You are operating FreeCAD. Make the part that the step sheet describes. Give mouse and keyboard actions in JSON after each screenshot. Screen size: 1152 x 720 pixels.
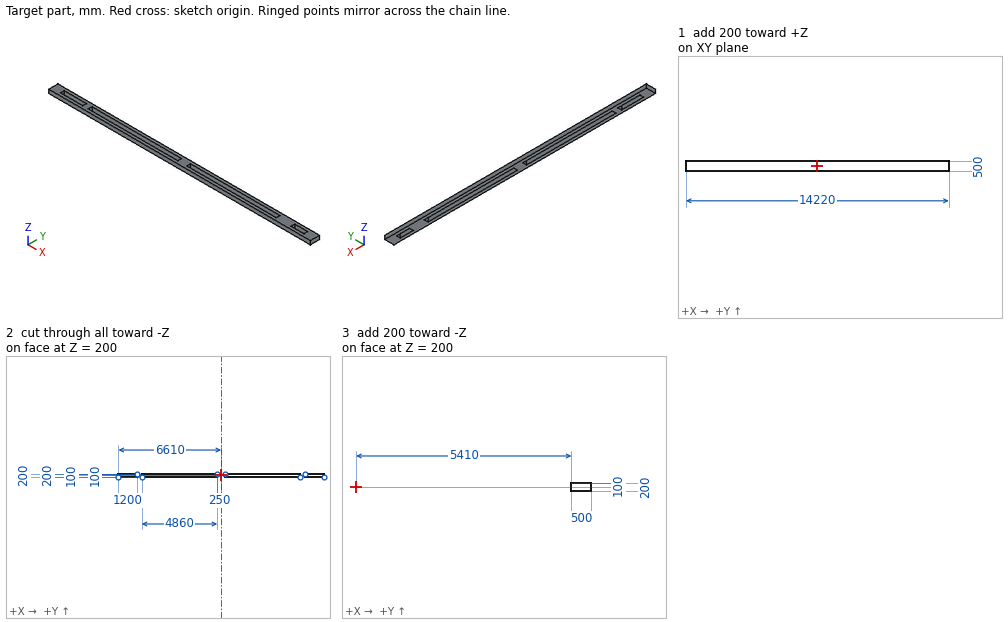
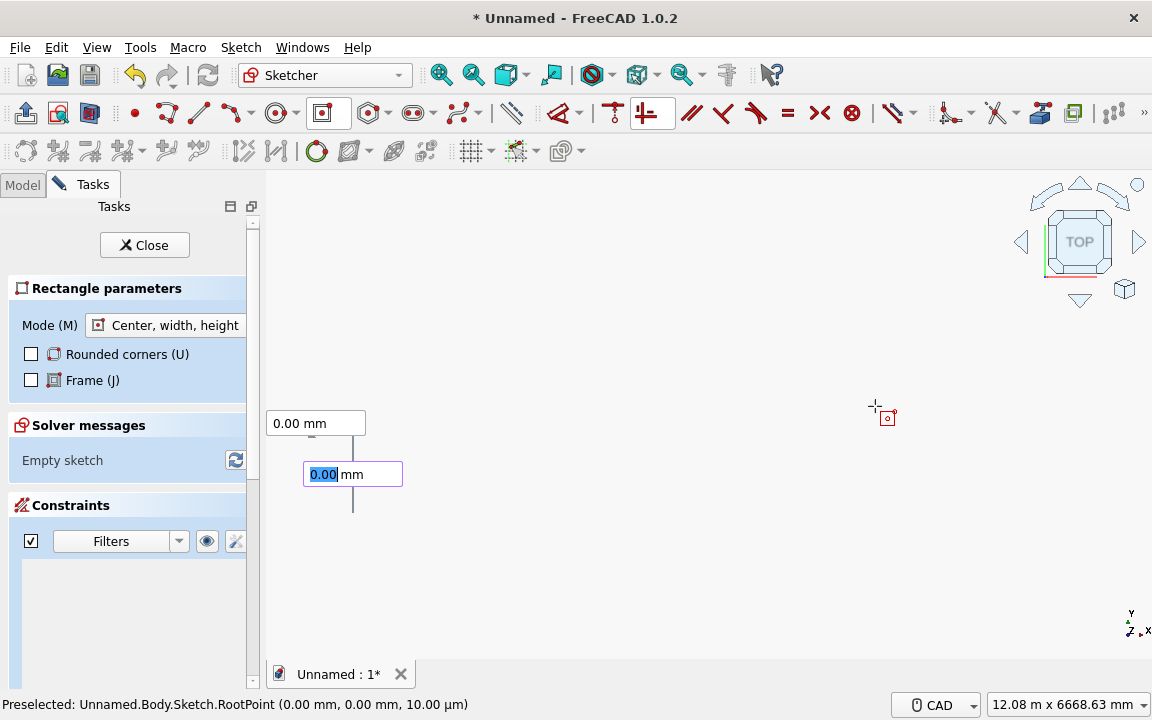
{"action": "left_click", "coordinate": [874, 406]}
{"action": "key", "text": "Escape"}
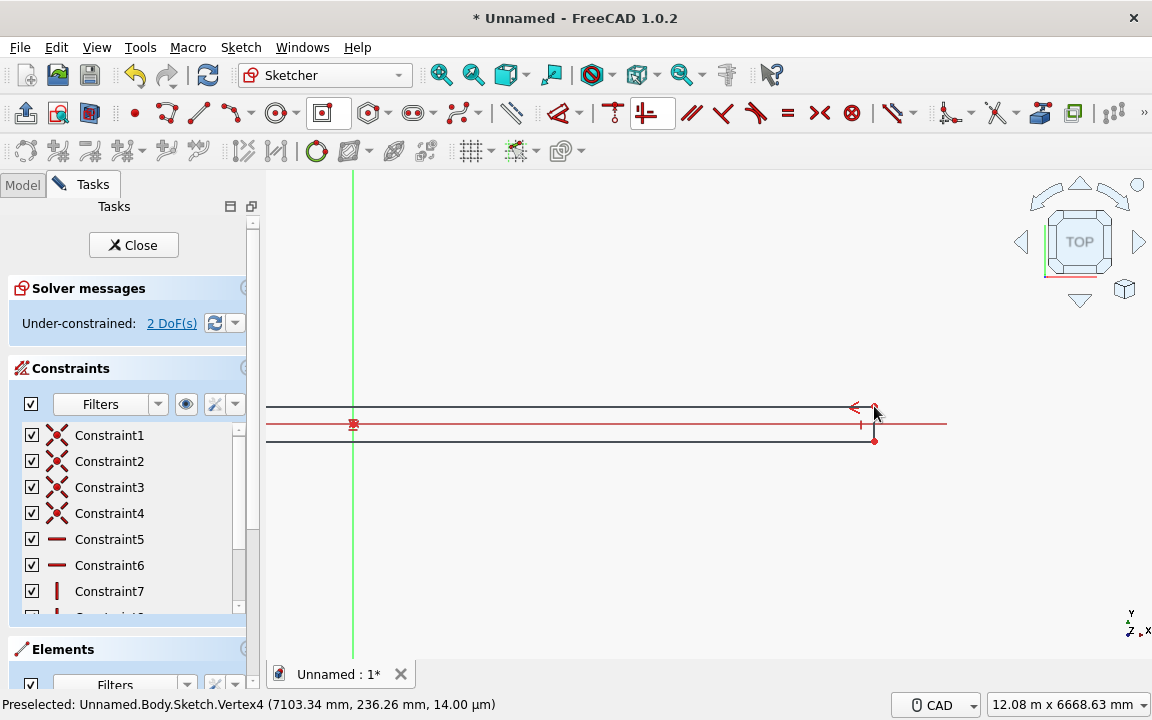
{"action": "left_click", "coordinate": [558, 114]}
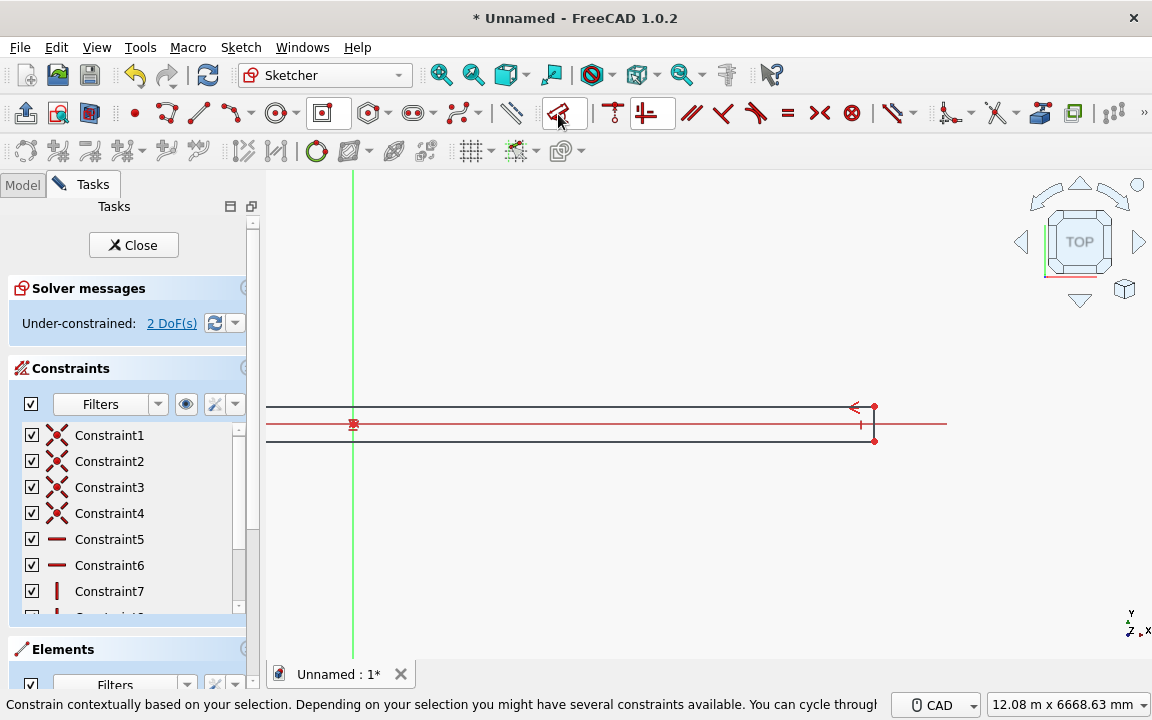
{"action": "left_click", "coordinate": [874, 428]}
{"action": "left_click", "coordinate": [908, 416]}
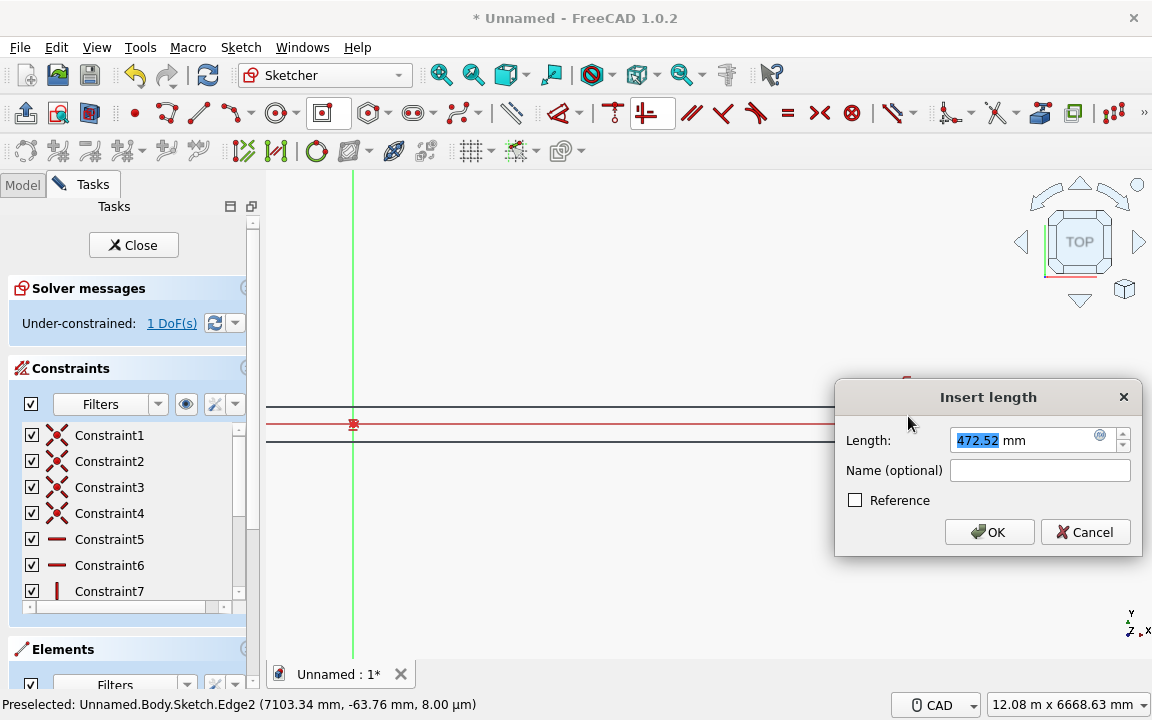
{"action": "type", "text": "500"}
{"action": "key", "text": "Return"}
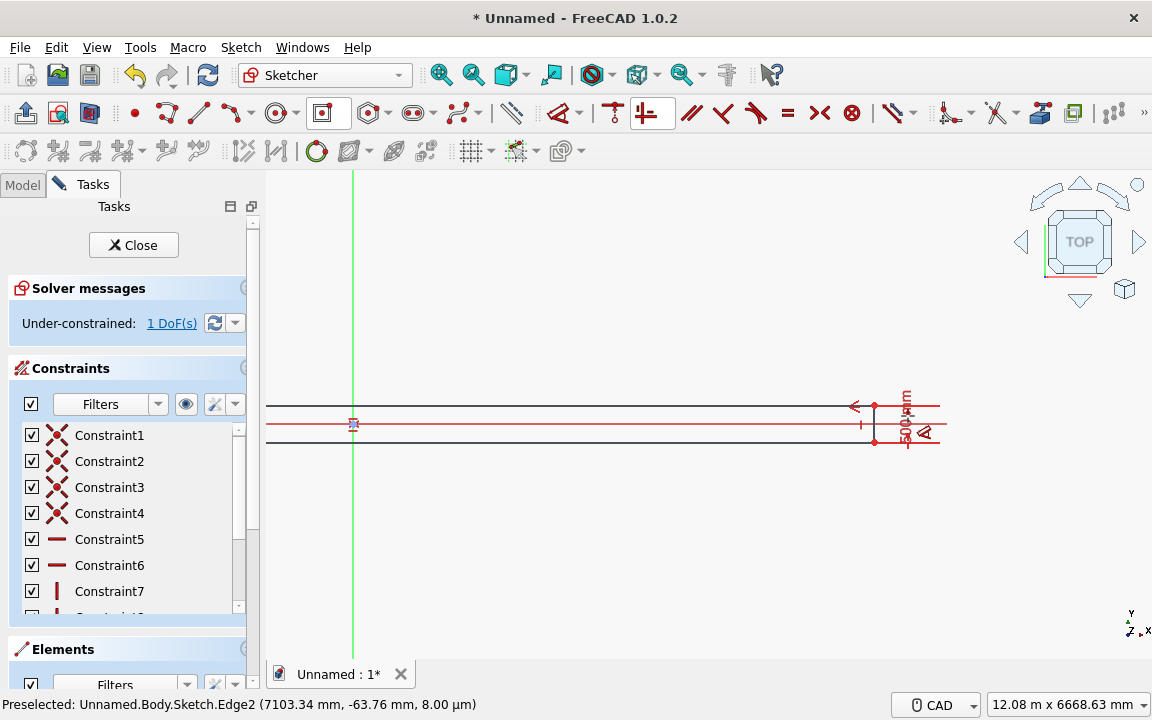
{"action": "left_click", "coordinate": [561, 443]}
{"action": "left_click", "coordinate": [584, 477]}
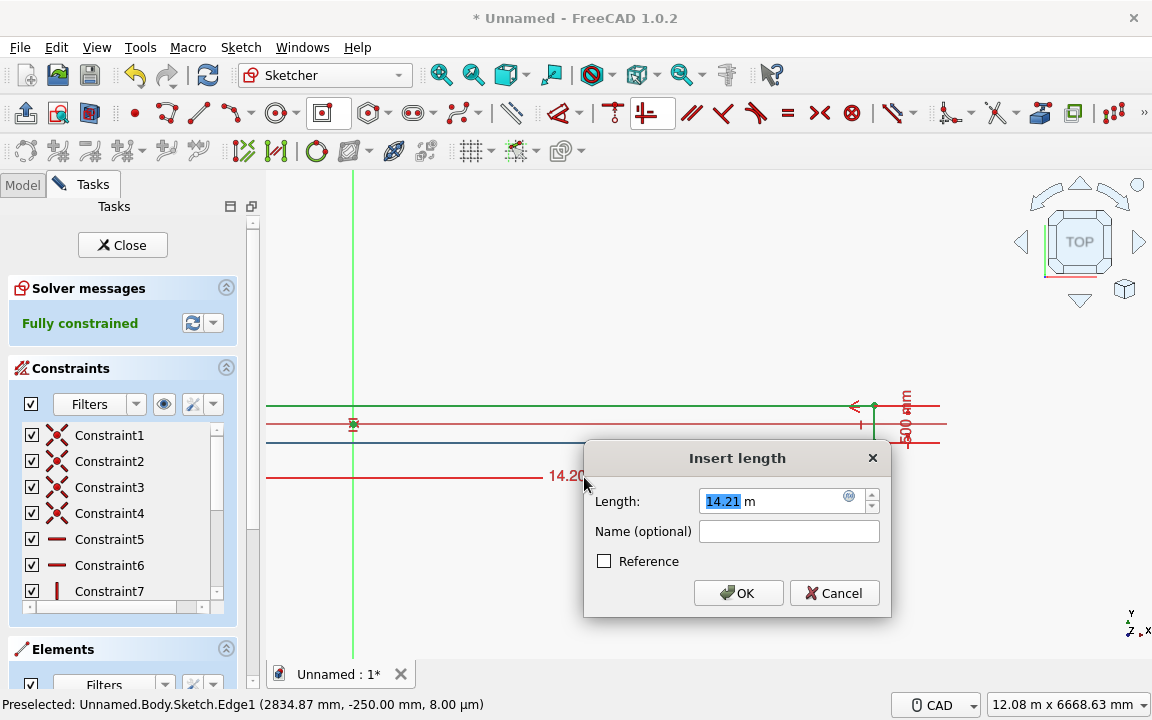
{"action": "key", "text": "ctrl+a"}
{"action": "type", "text": "14220 mm"}
{"action": "key", "text": "Return"}
{"action": "key", "text": "Escape"}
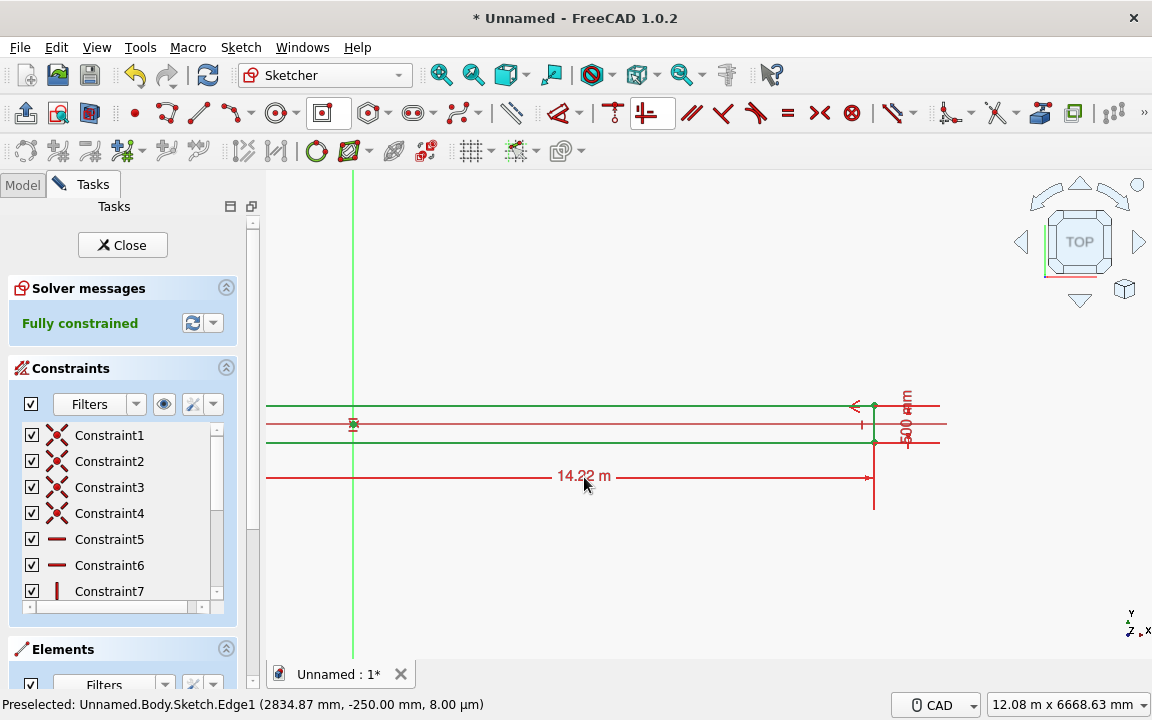
{"action": "left_click", "coordinate": [123, 245]}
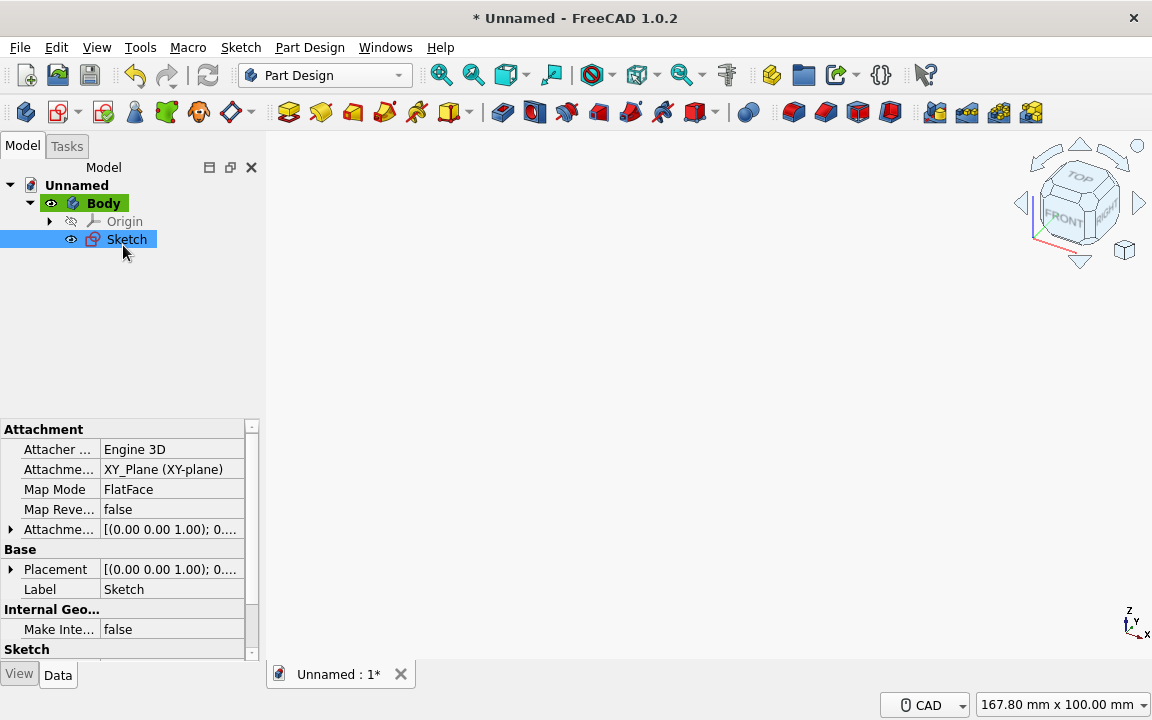
{"action": "left_click", "coordinate": [290, 112]}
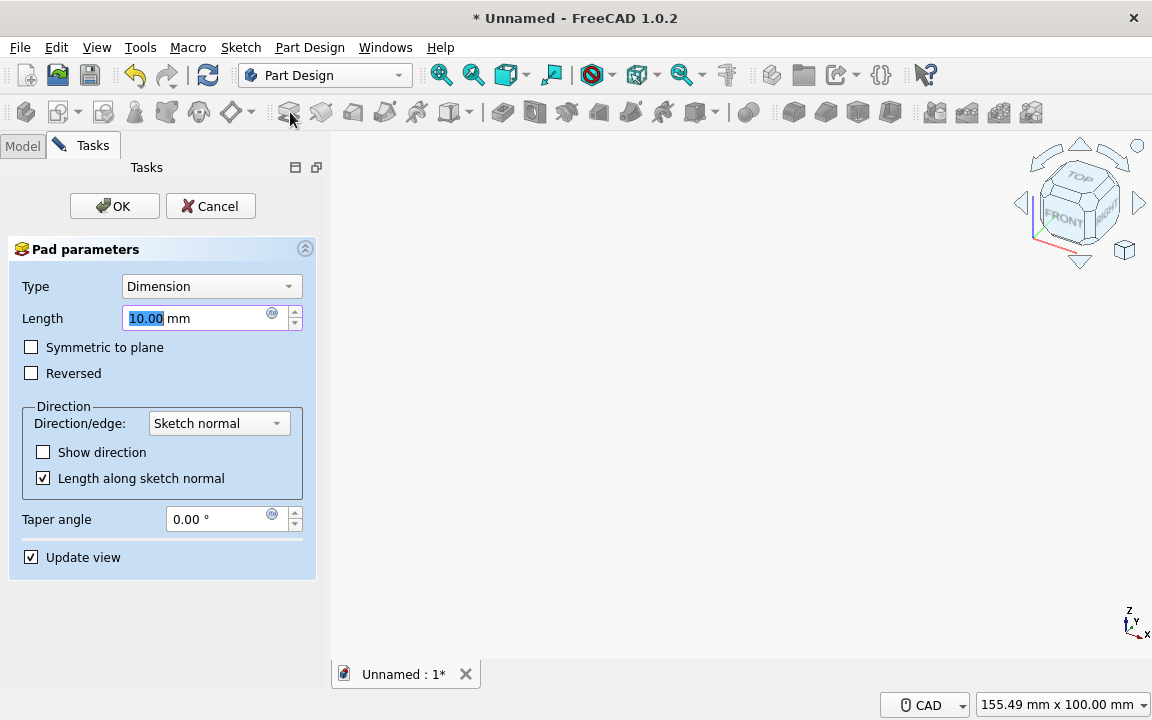
{"action": "type", "text": "200"}
{"action": "key", "text": "Tab"}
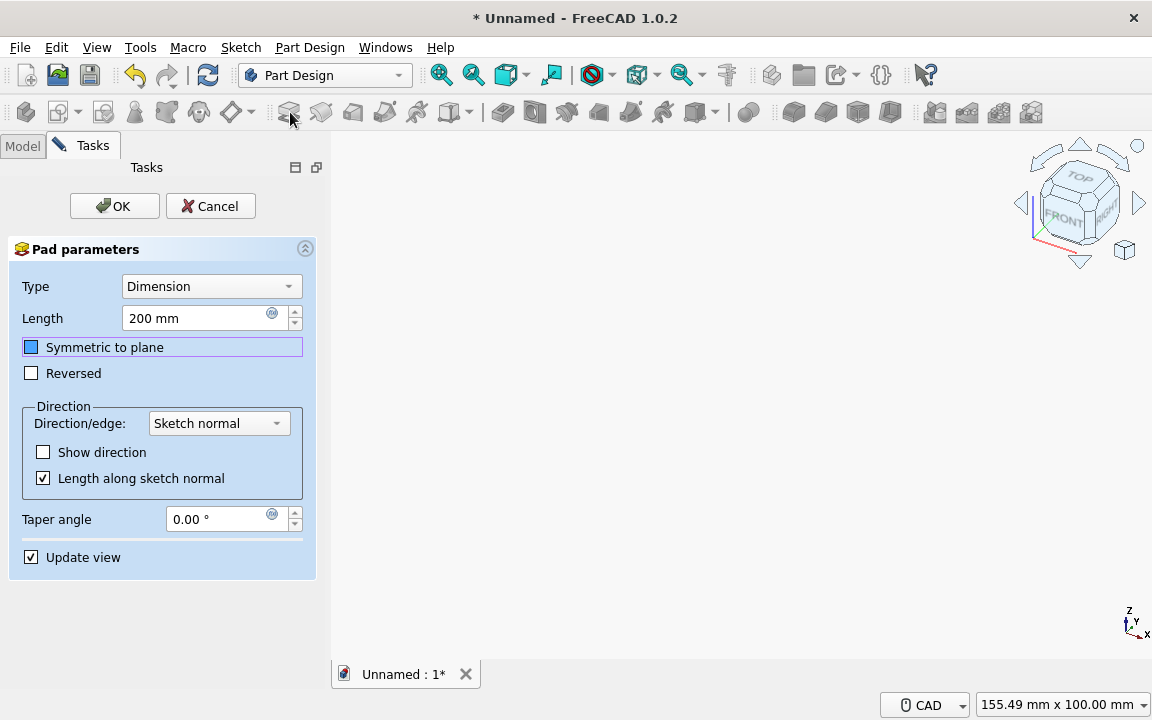
{"action": "left_click", "coordinate": [115, 206]}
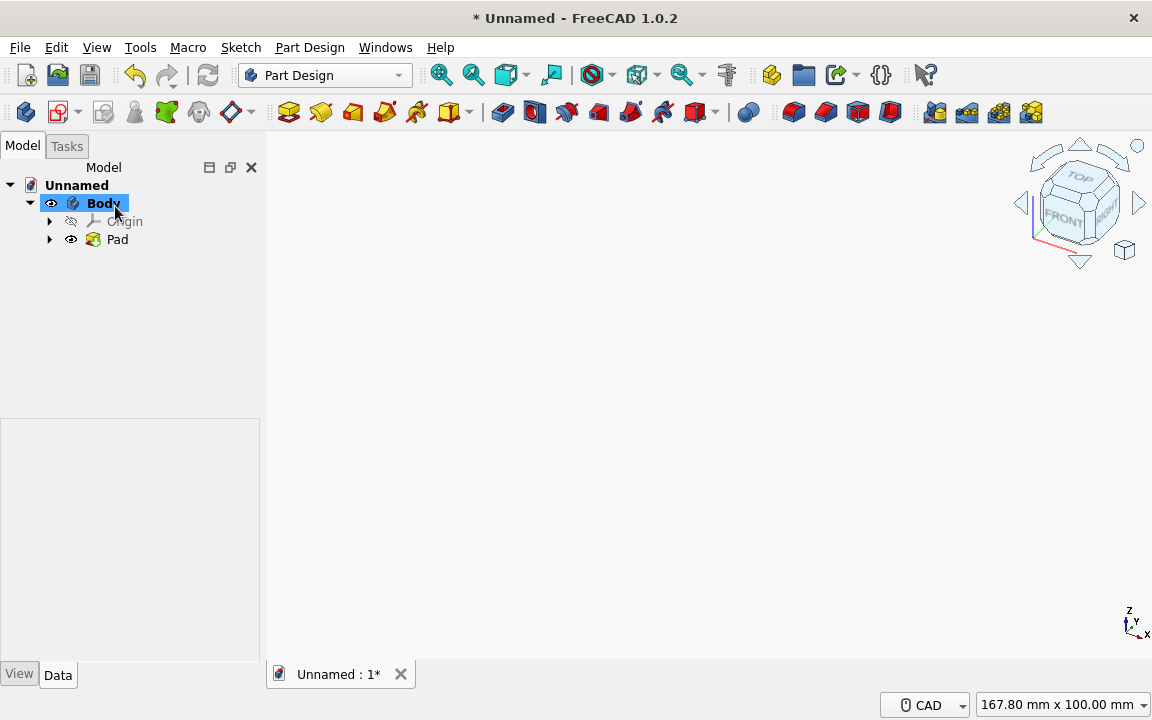
{"action": "left_click", "coordinate": [442, 76]}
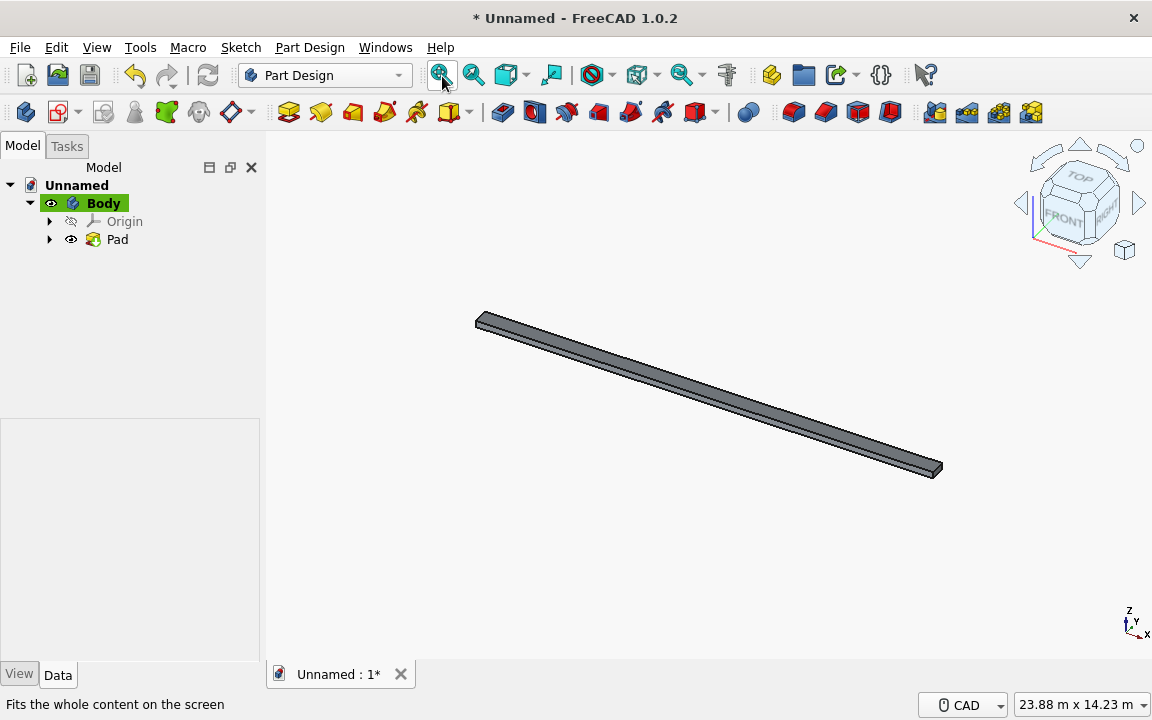
{"action": "key", "text": "0"}